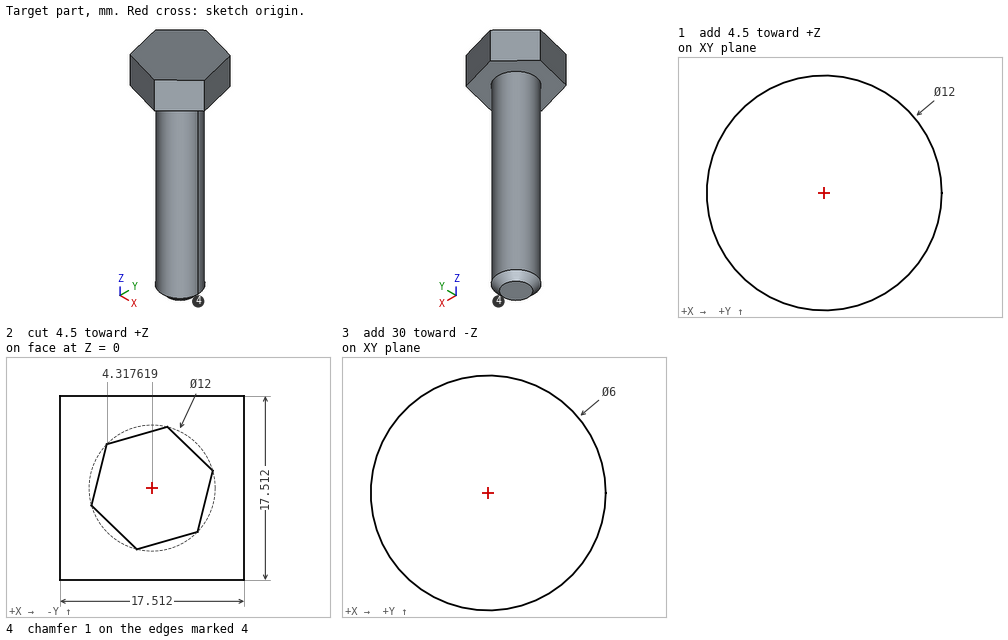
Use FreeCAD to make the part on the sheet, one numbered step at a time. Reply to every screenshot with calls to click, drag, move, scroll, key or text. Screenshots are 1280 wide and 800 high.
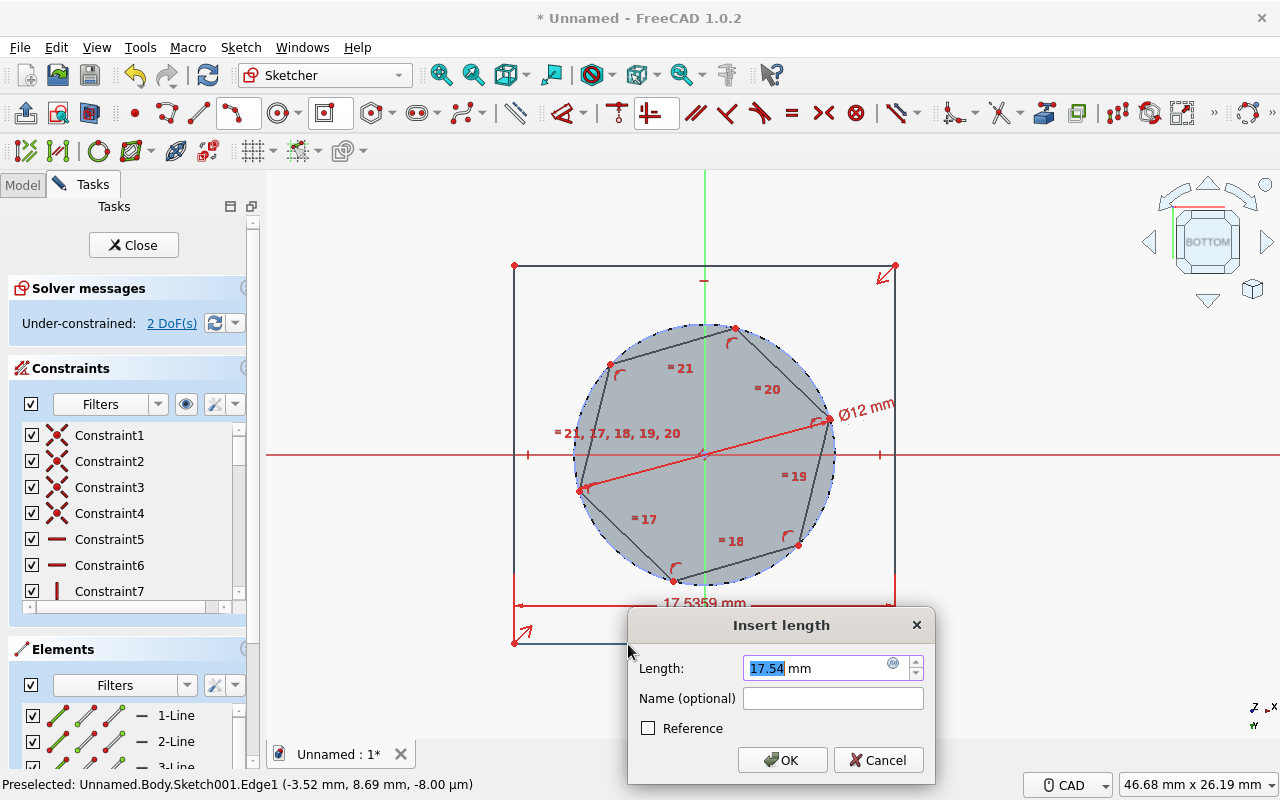
text(17.512)
key(Return)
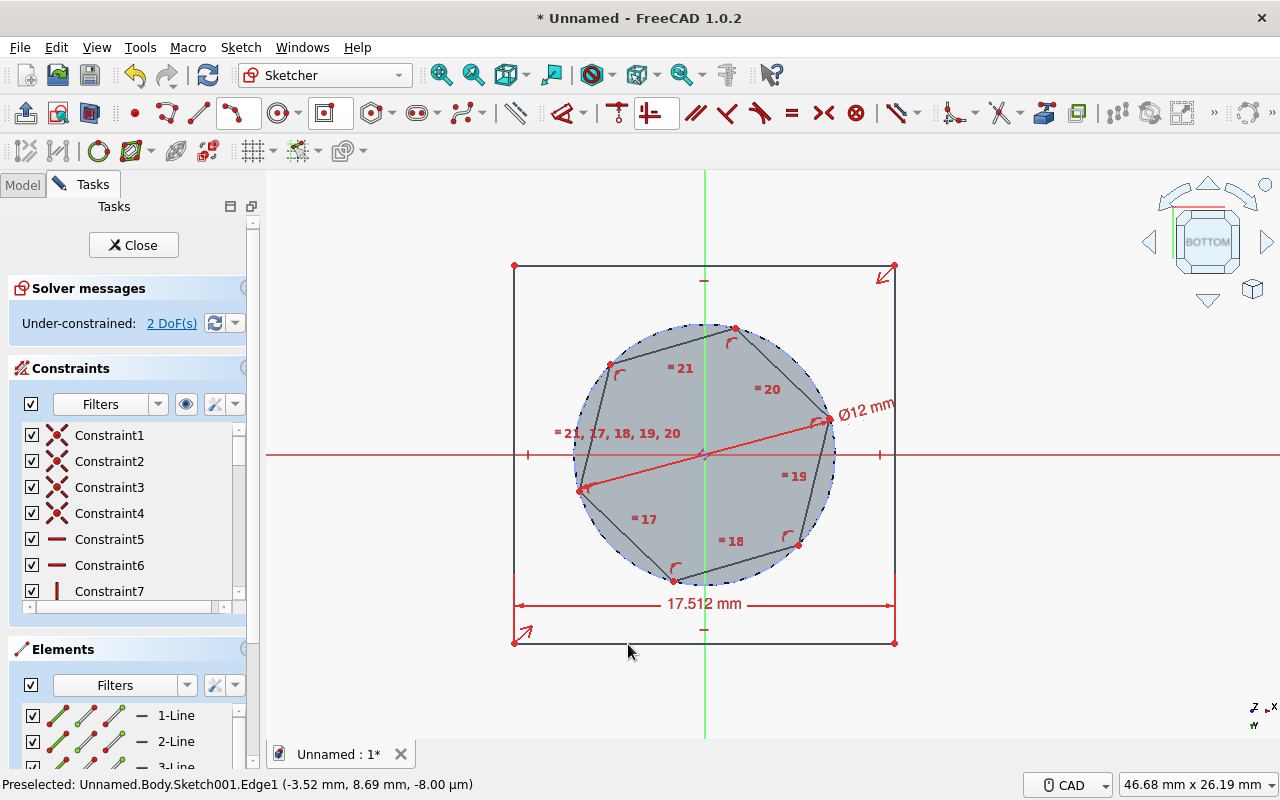
click(895, 530)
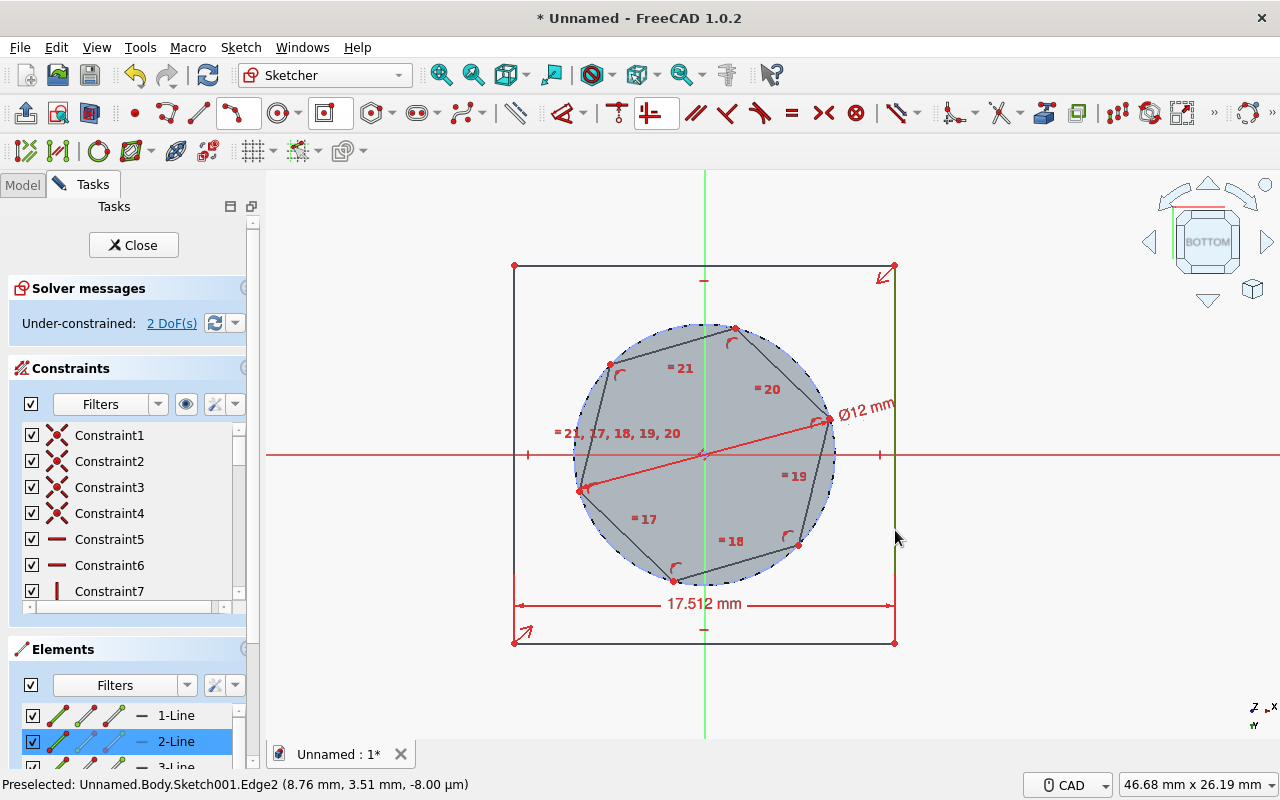
key(i)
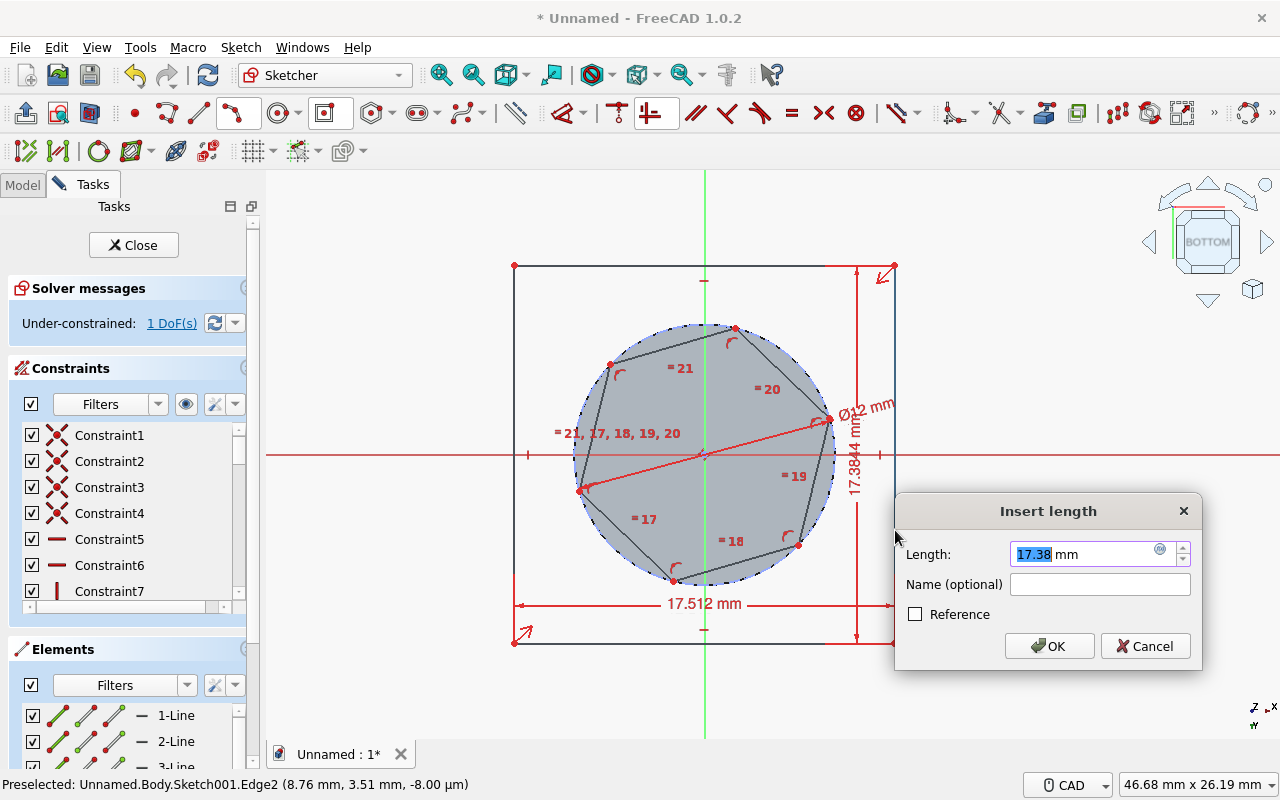
text(17.512)
key(Return)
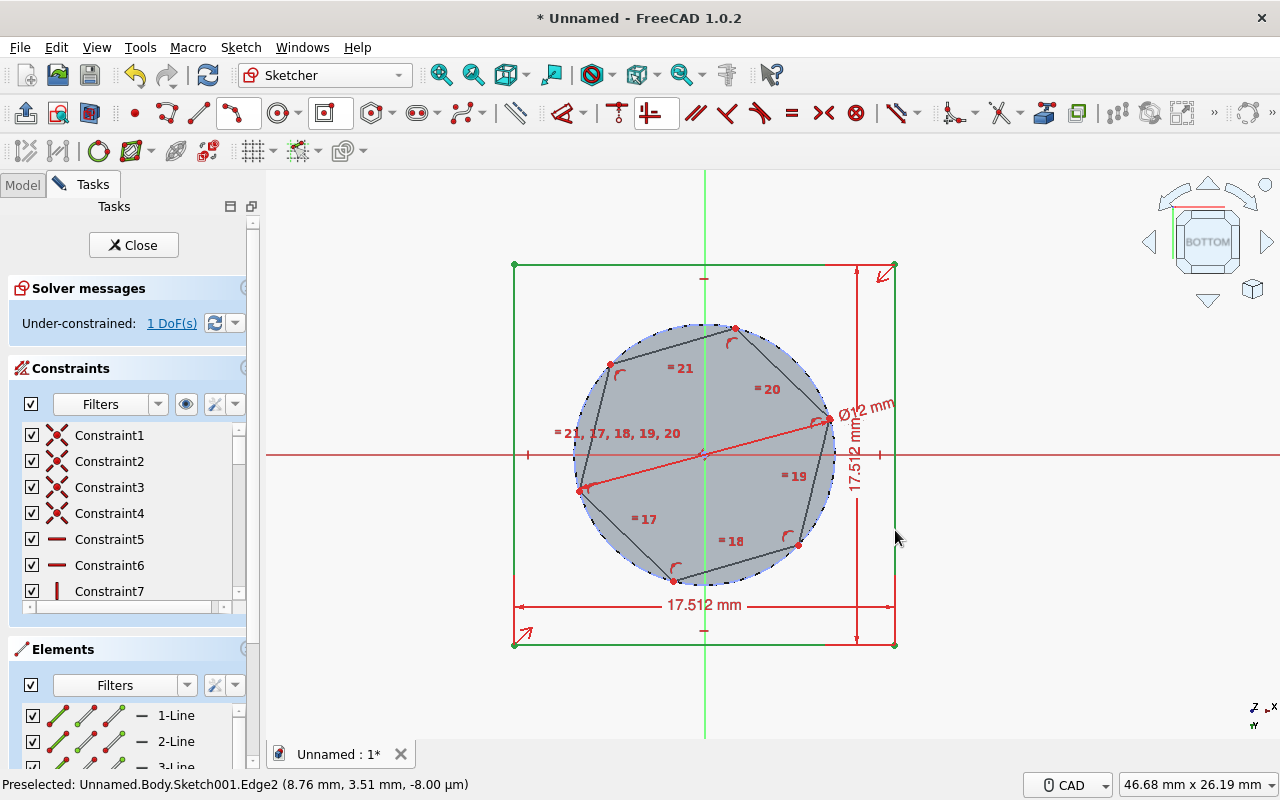
click(610, 365)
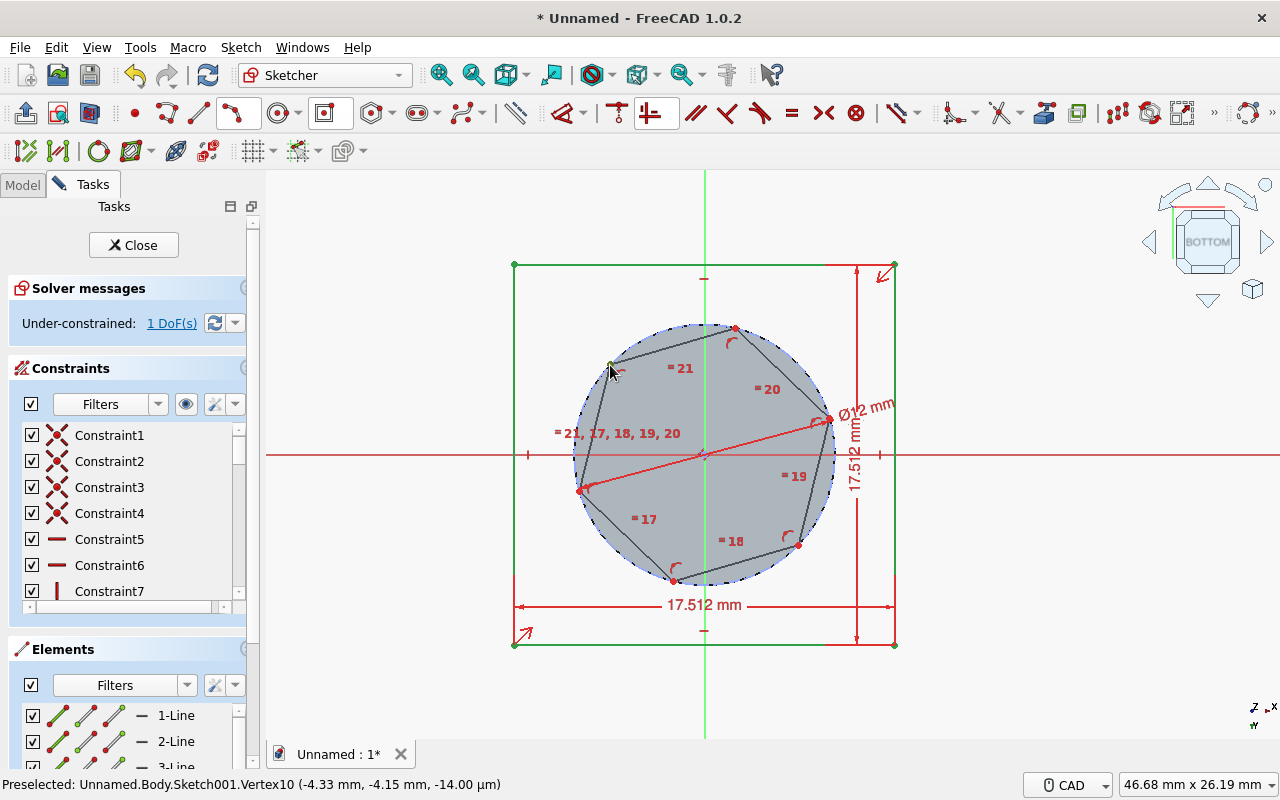
click(586, 114)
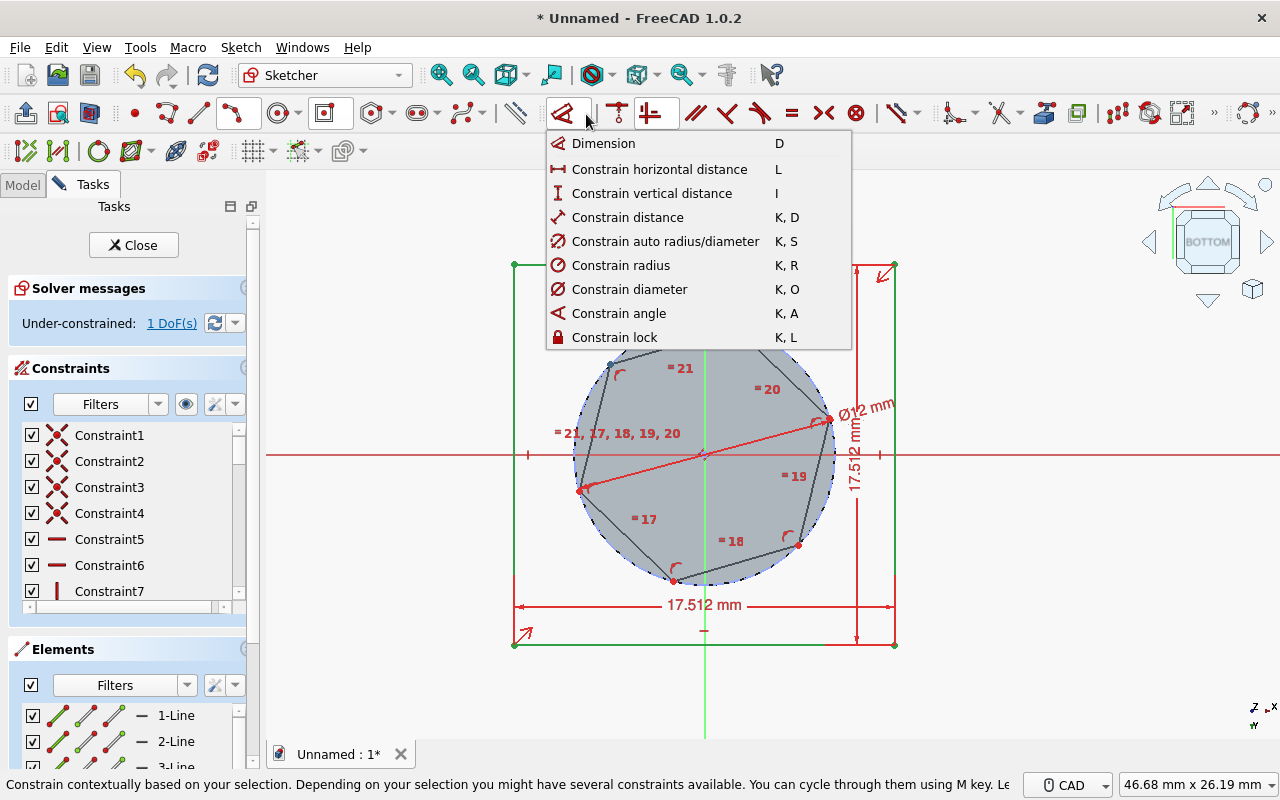
click(699, 169)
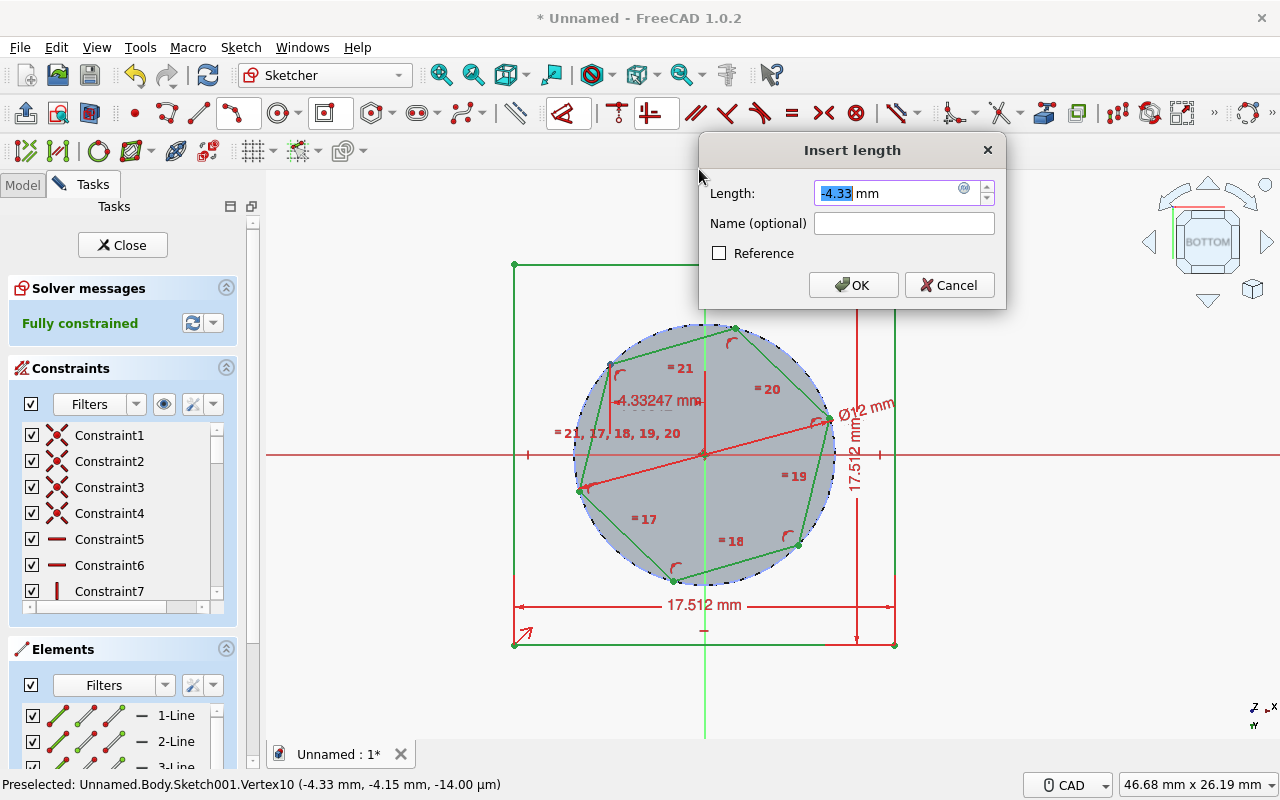
text(-4.317619)
key(Return)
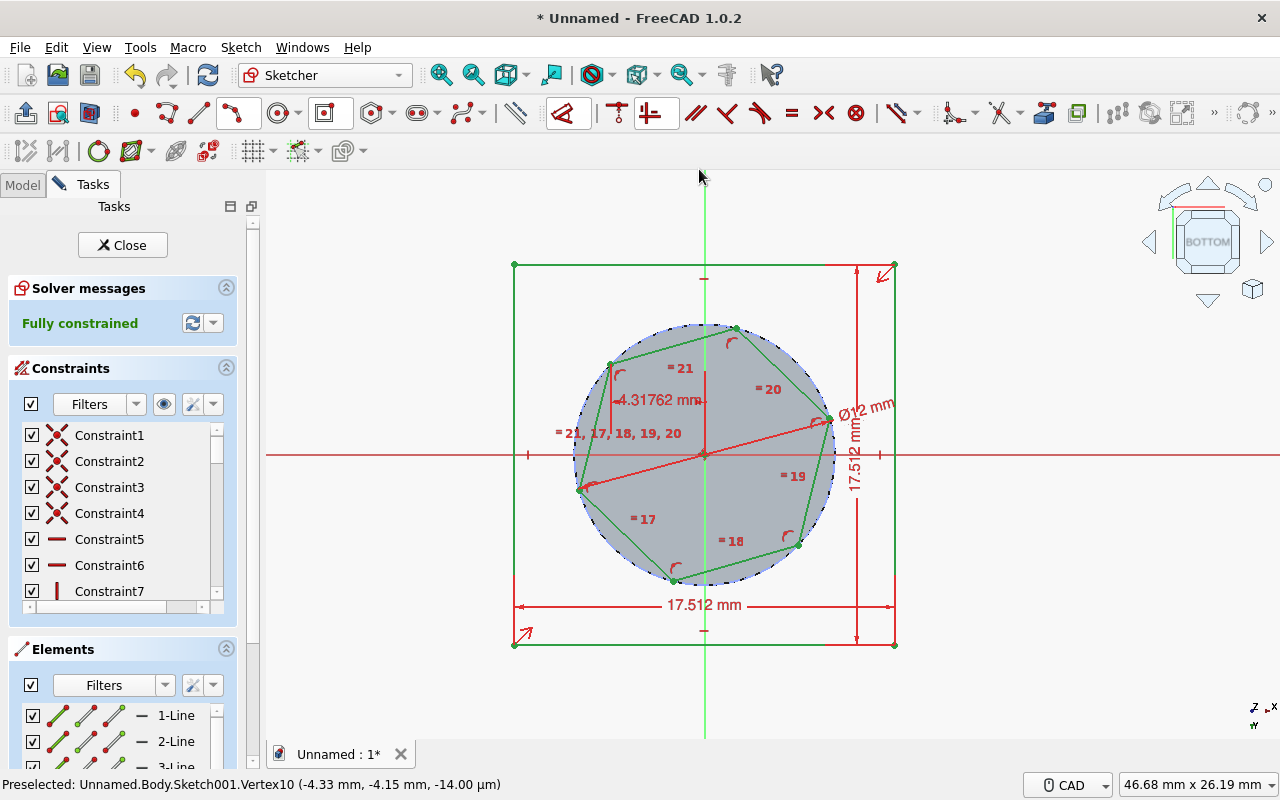
click(123, 245)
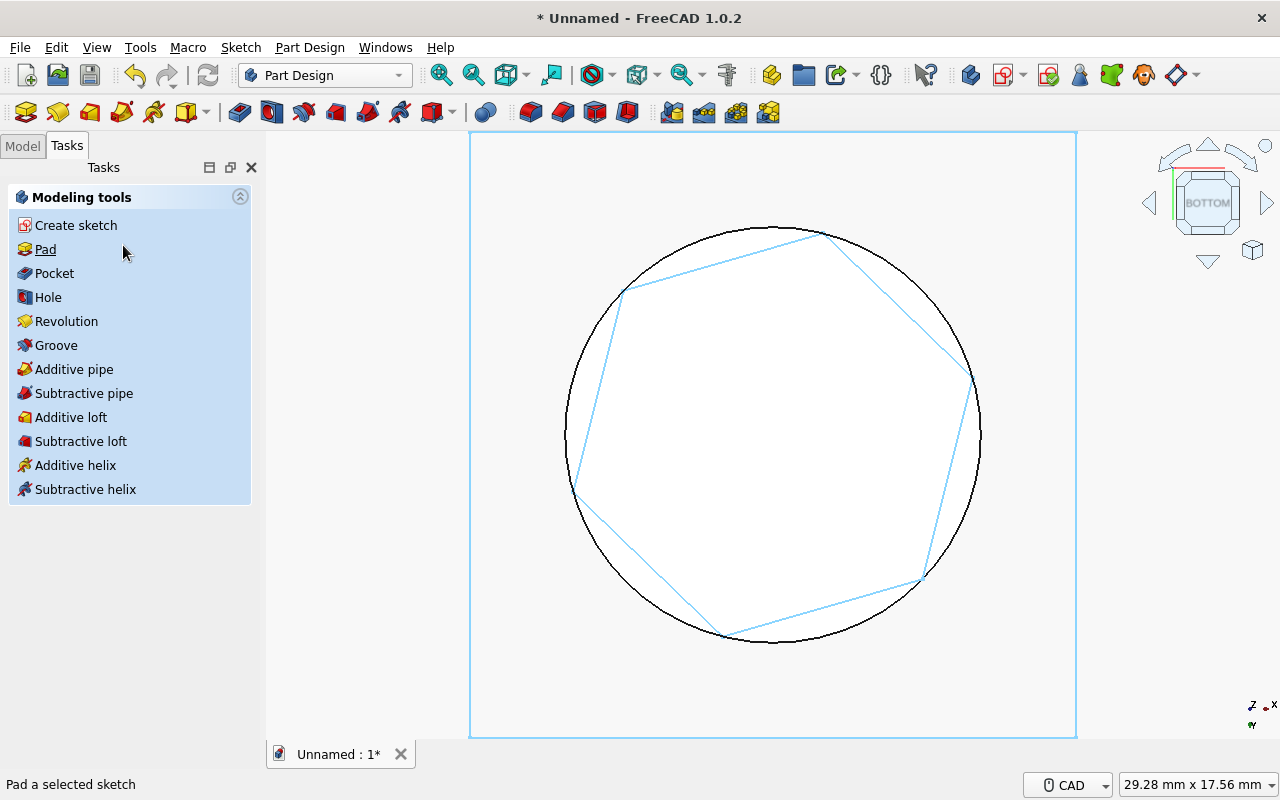
click(240, 112)